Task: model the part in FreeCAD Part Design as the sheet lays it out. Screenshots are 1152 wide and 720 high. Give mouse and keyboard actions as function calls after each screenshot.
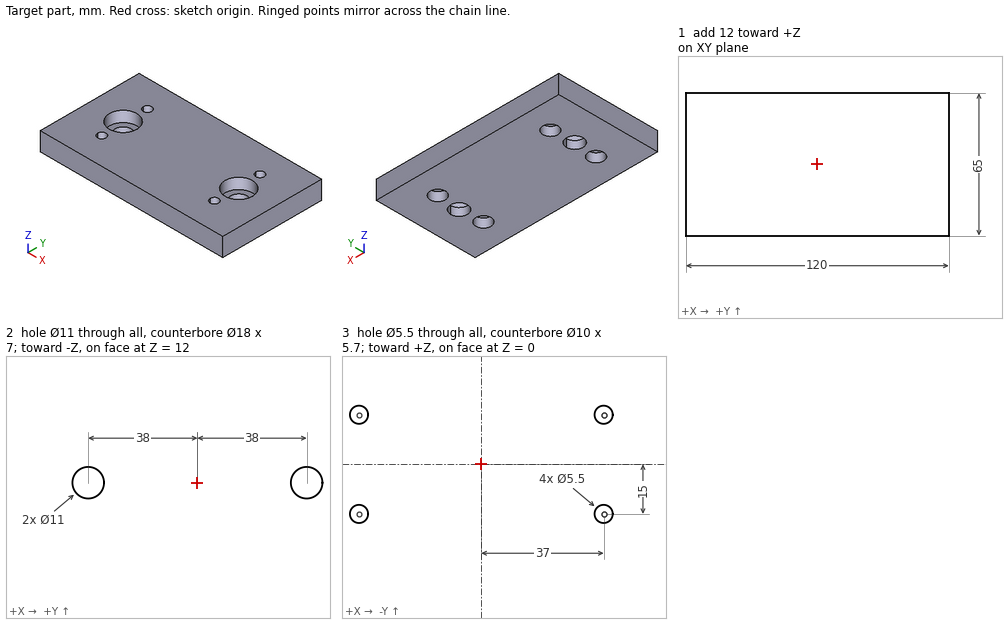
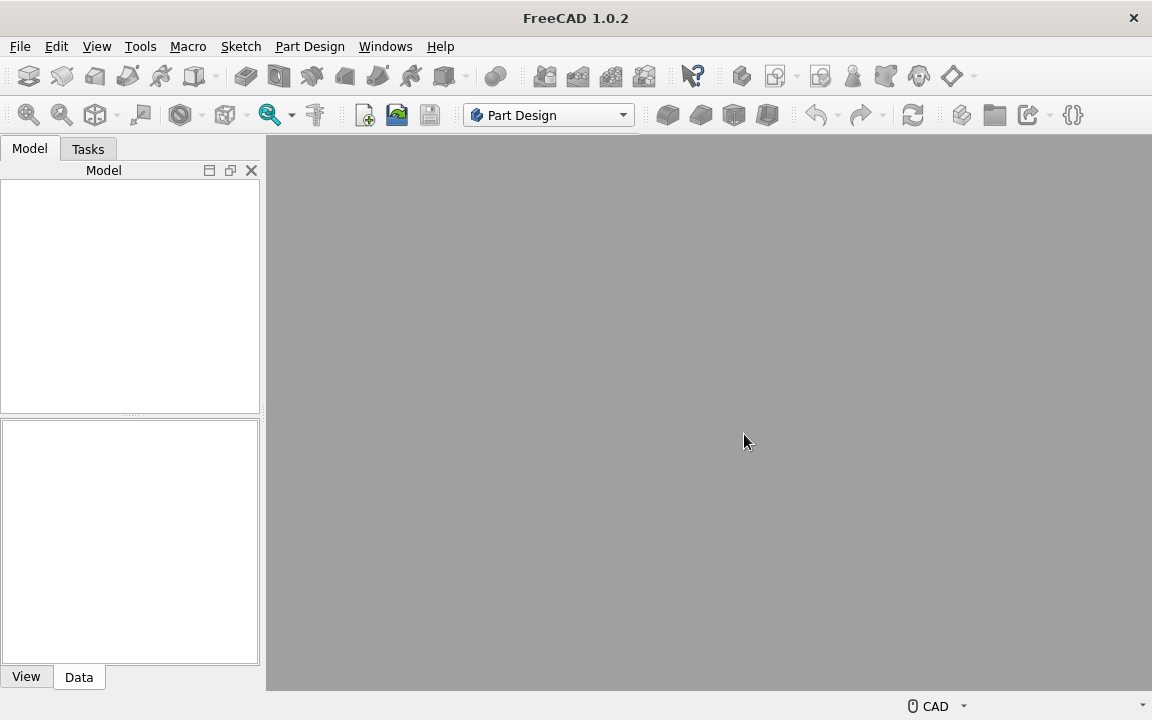
click(364, 116)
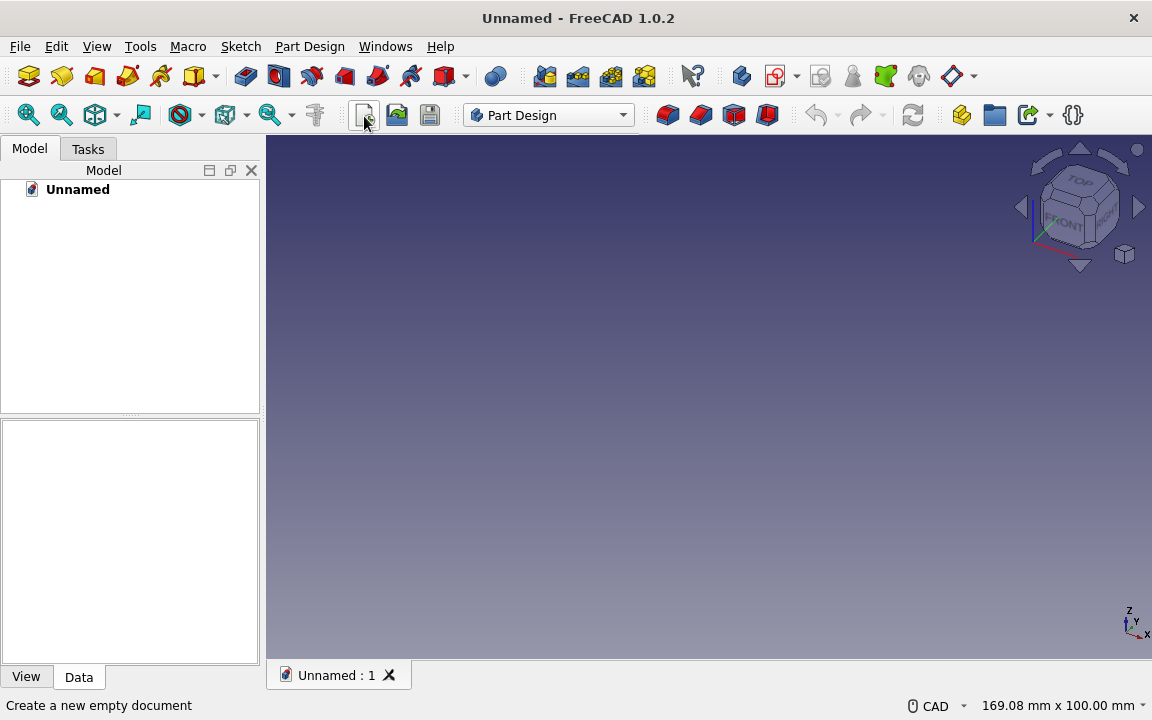
click(774, 76)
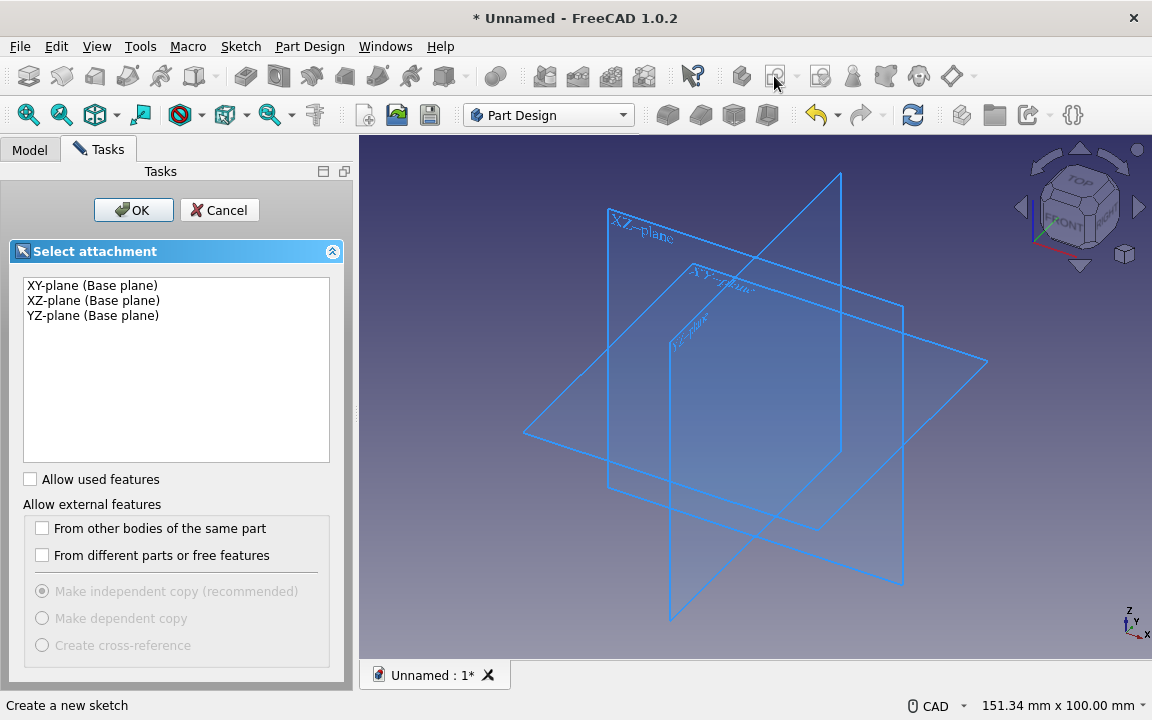
click(84, 286)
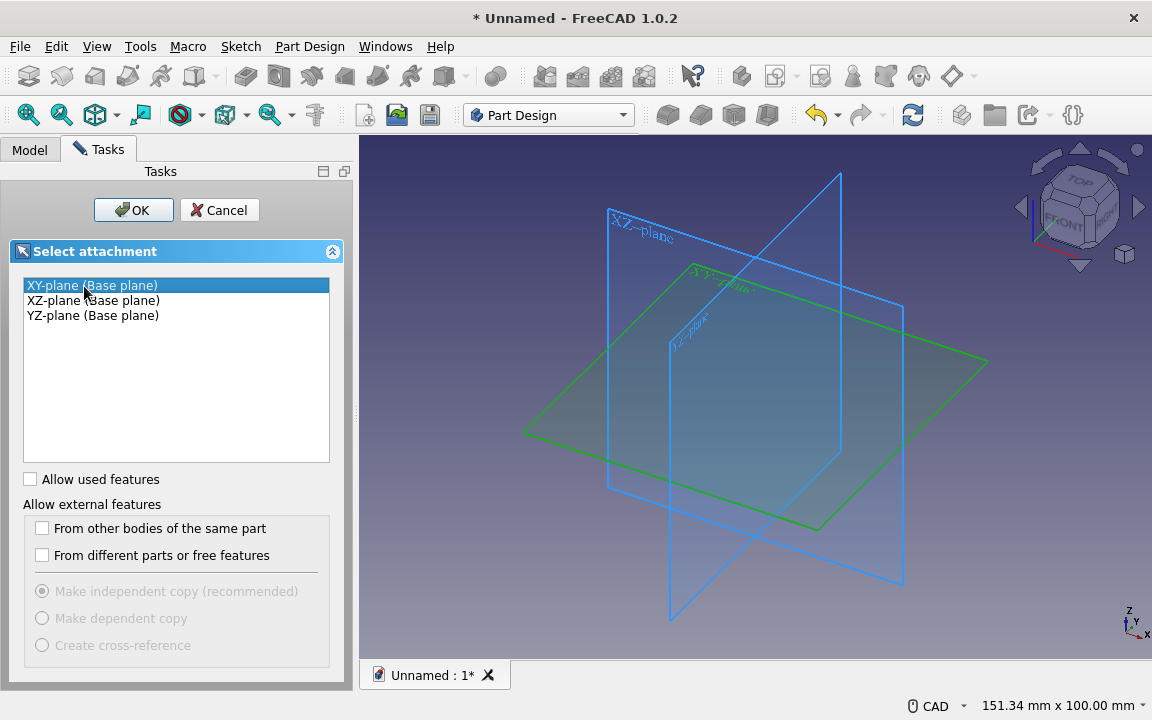
click(134, 210)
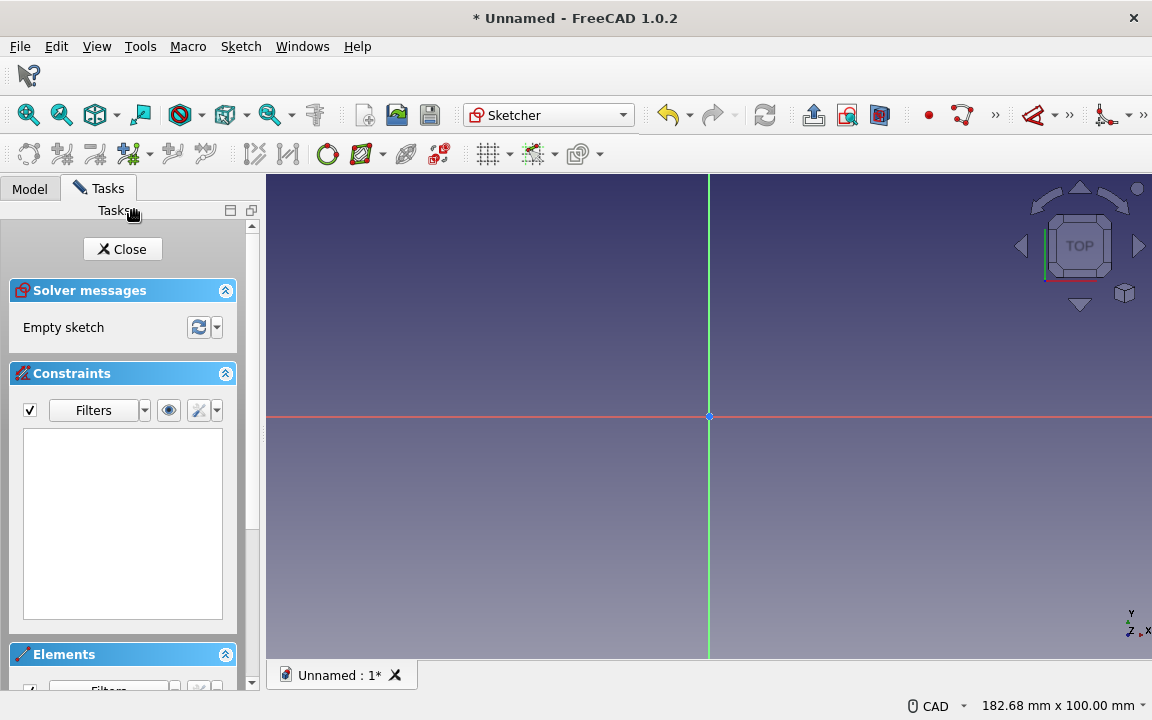
scroll(331, 416, down, 1)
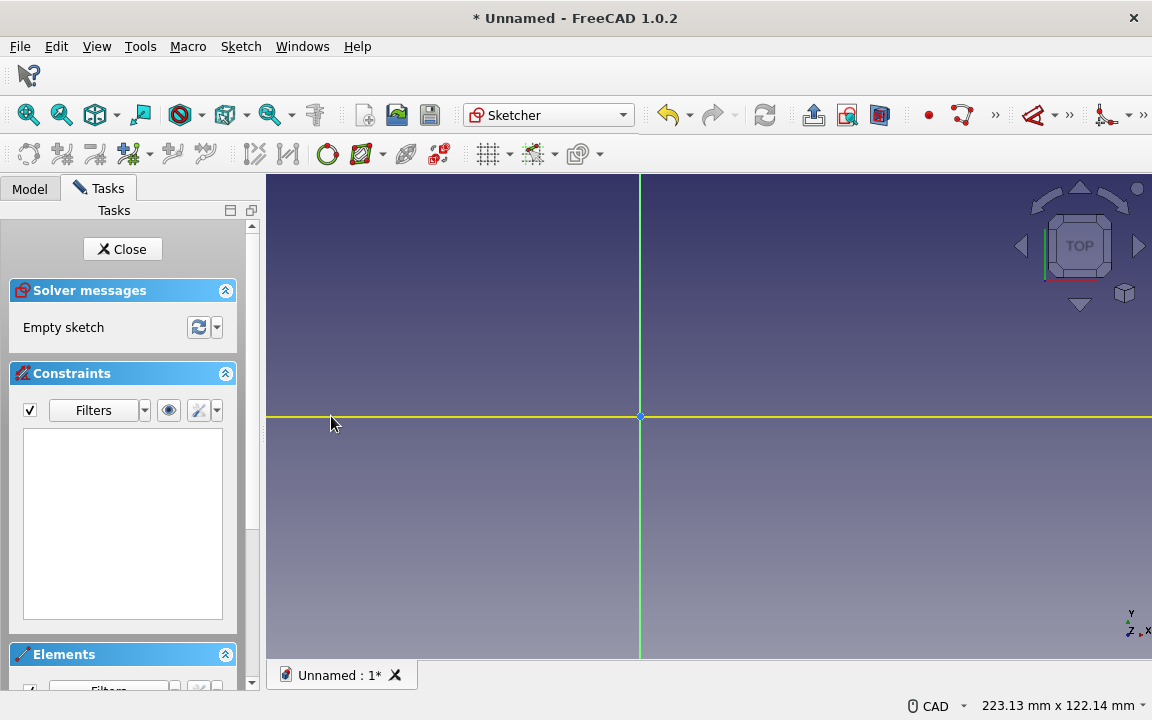
key(g)
key(v)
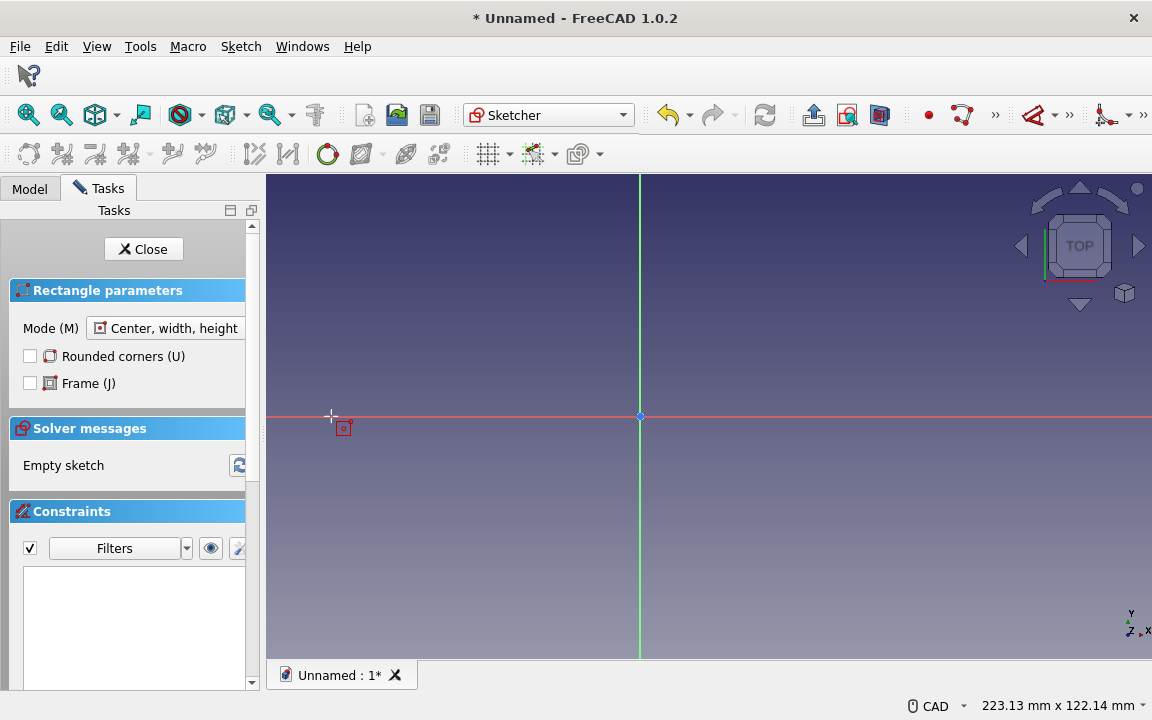
click(640, 416)
move(879, 287)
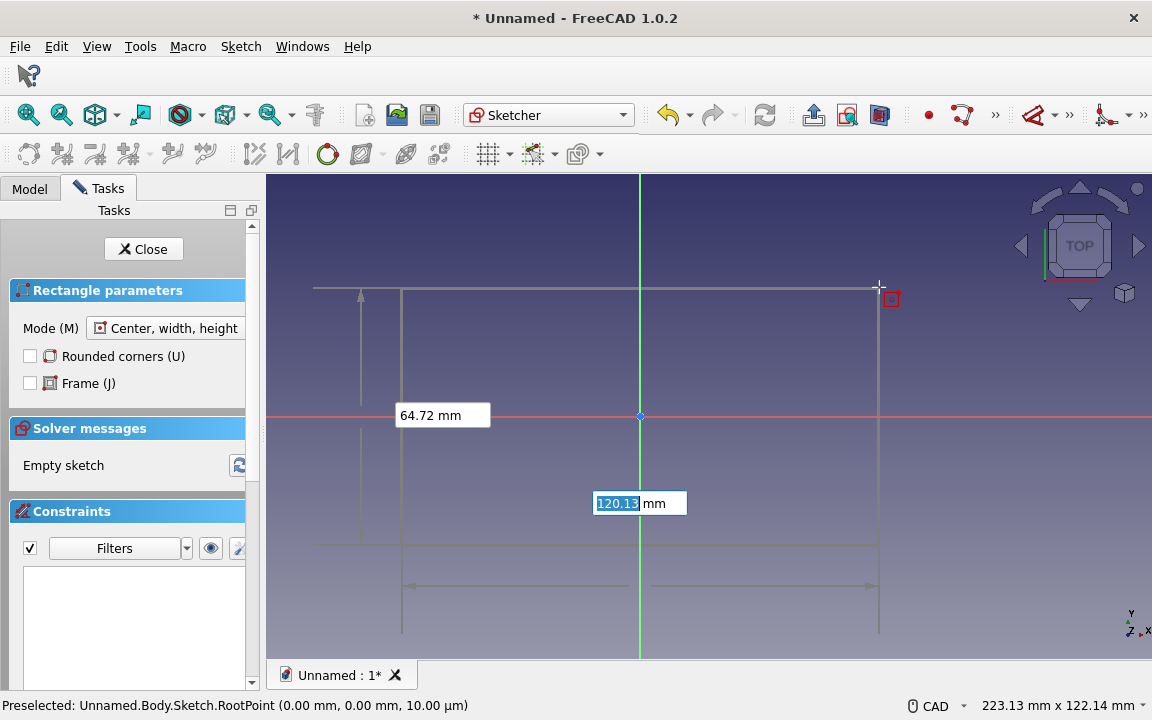
text(120)
key(Tab)
text(65)
key(Return)
key(Escape)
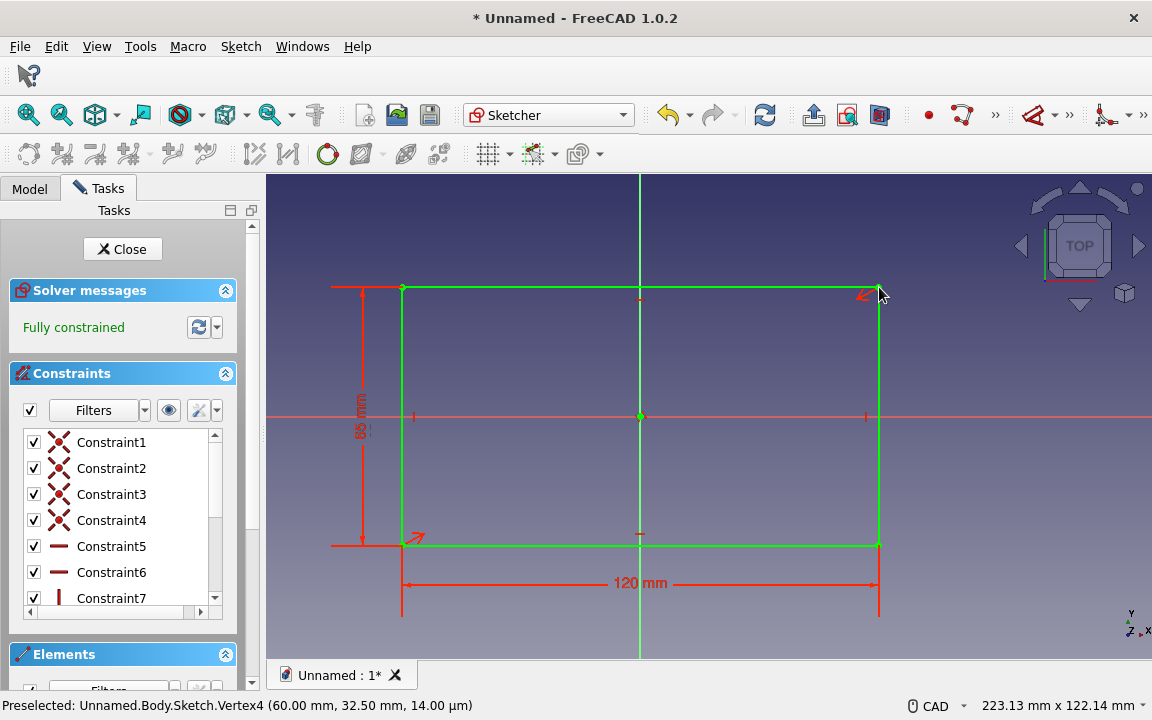
click(123, 249)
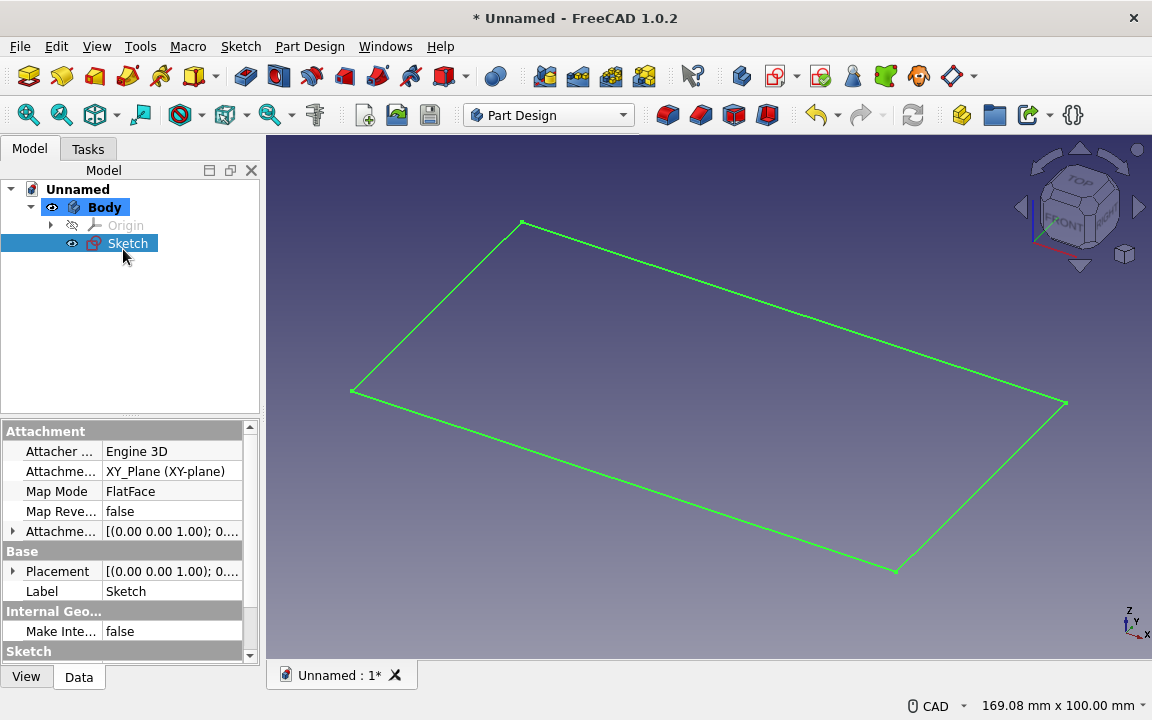
click(29, 76)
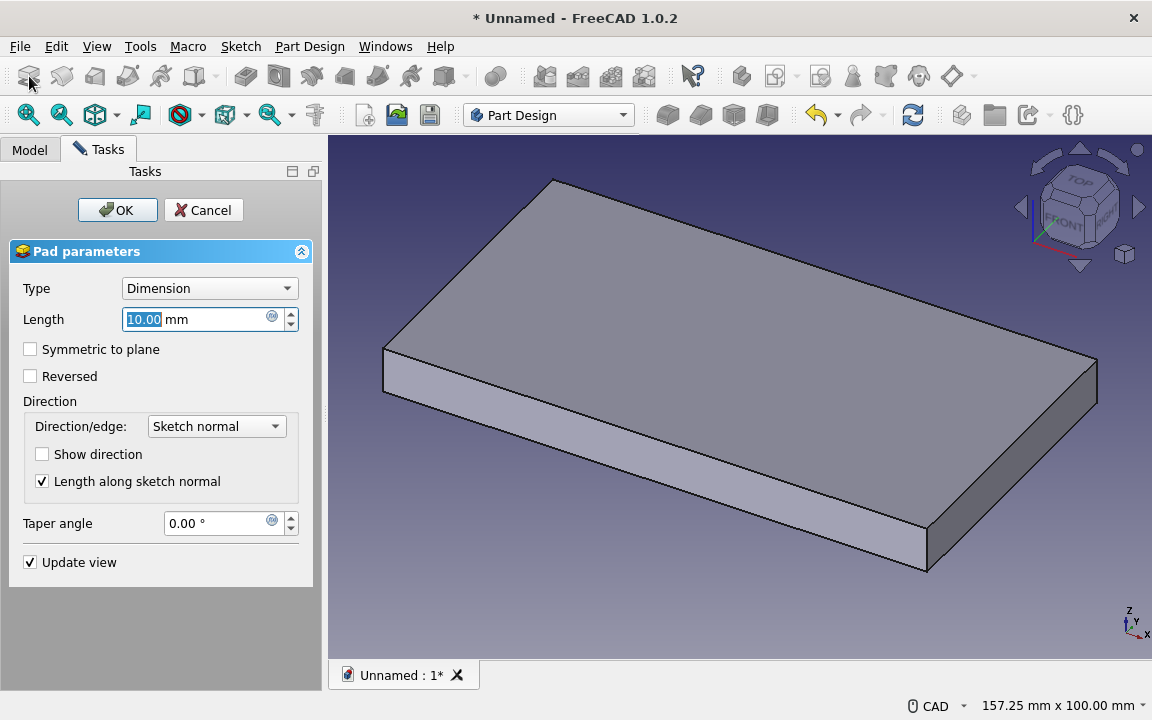
text(12)
key(Tab)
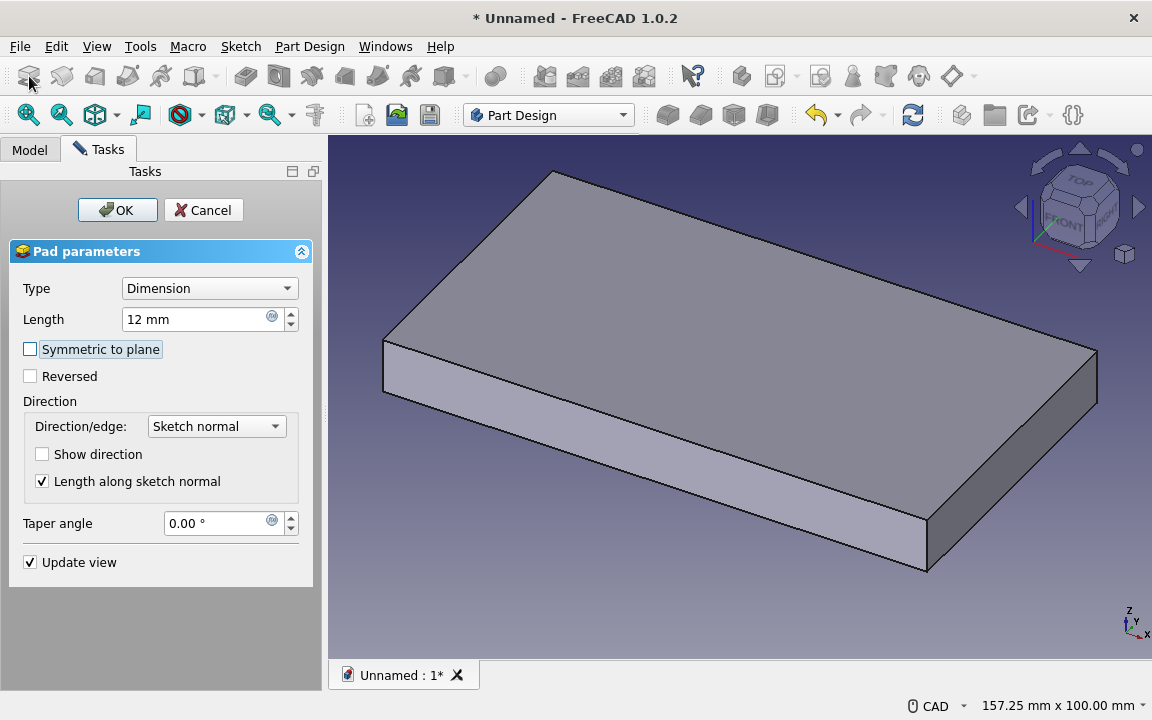
click(118, 210)